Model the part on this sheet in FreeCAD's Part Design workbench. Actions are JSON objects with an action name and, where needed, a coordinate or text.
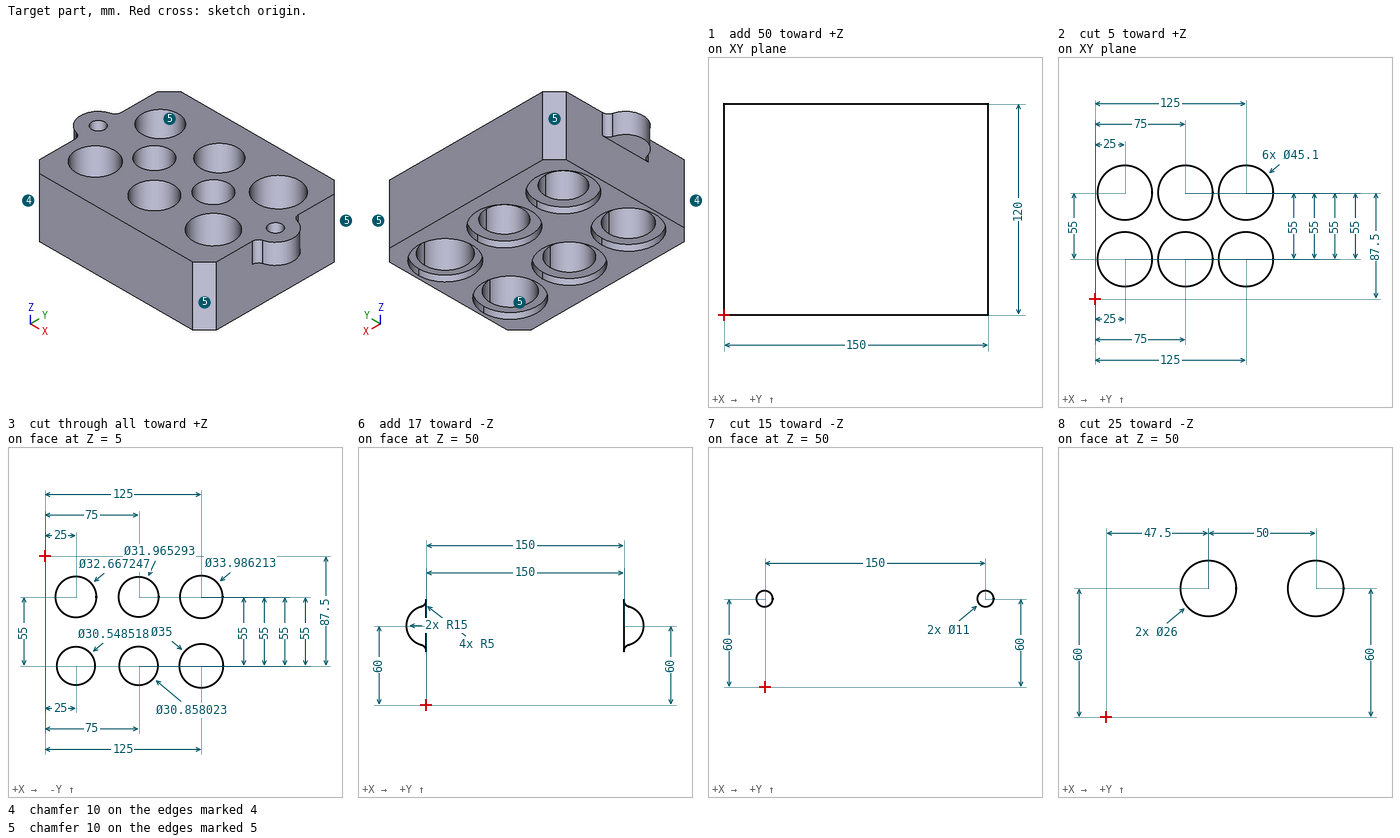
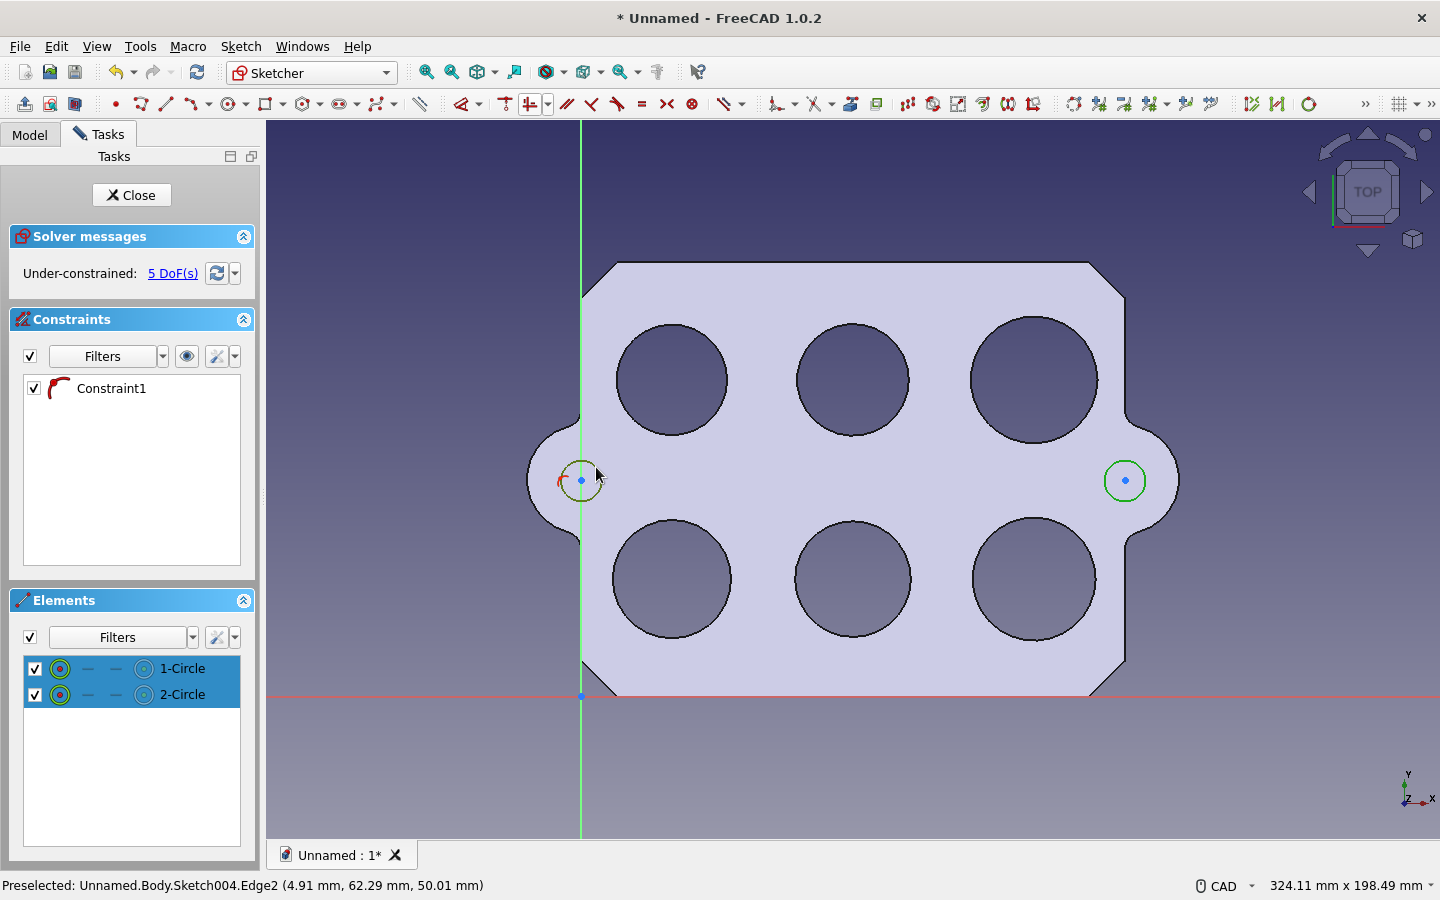
{"action": "left_click", "coordinate": [642, 104]}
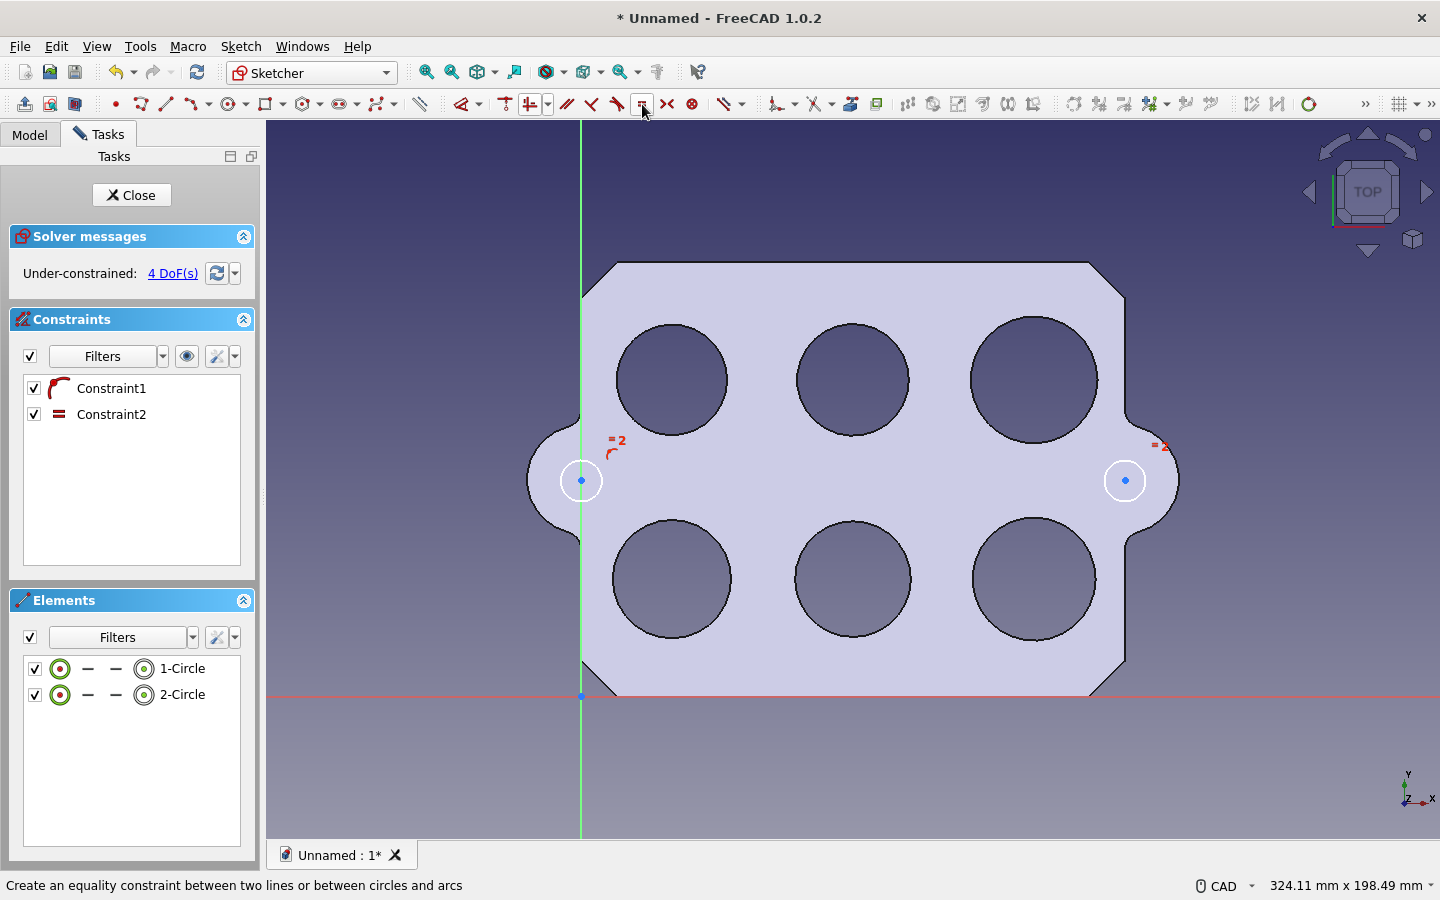
{"action": "key", "text": "d"}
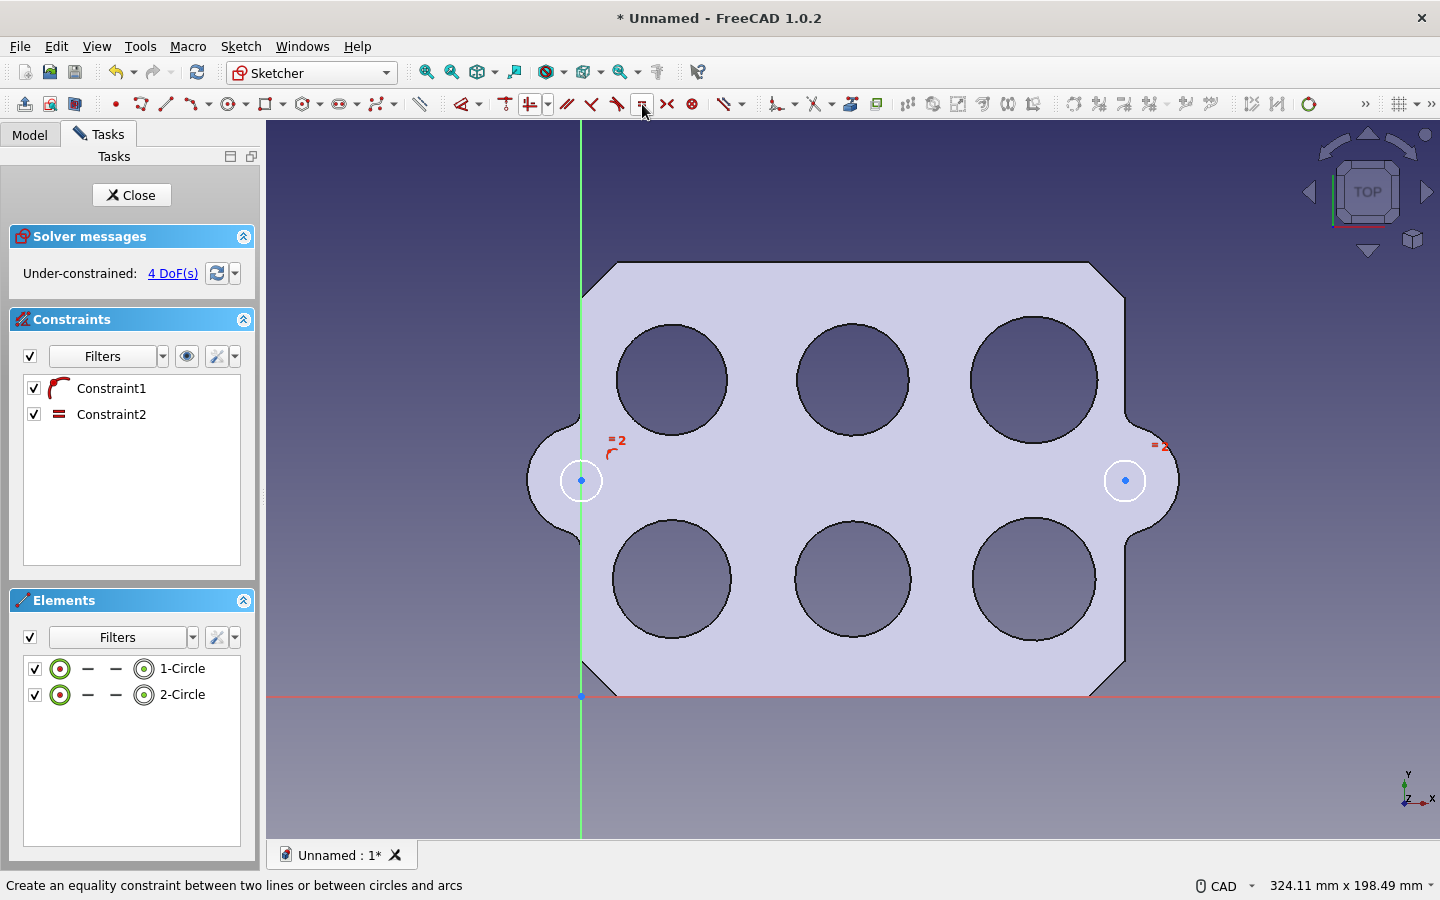
{"action": "left_click", "coordinate": [1139, 466]}
{"action": "left_click", "coordinate": [1161, 443]}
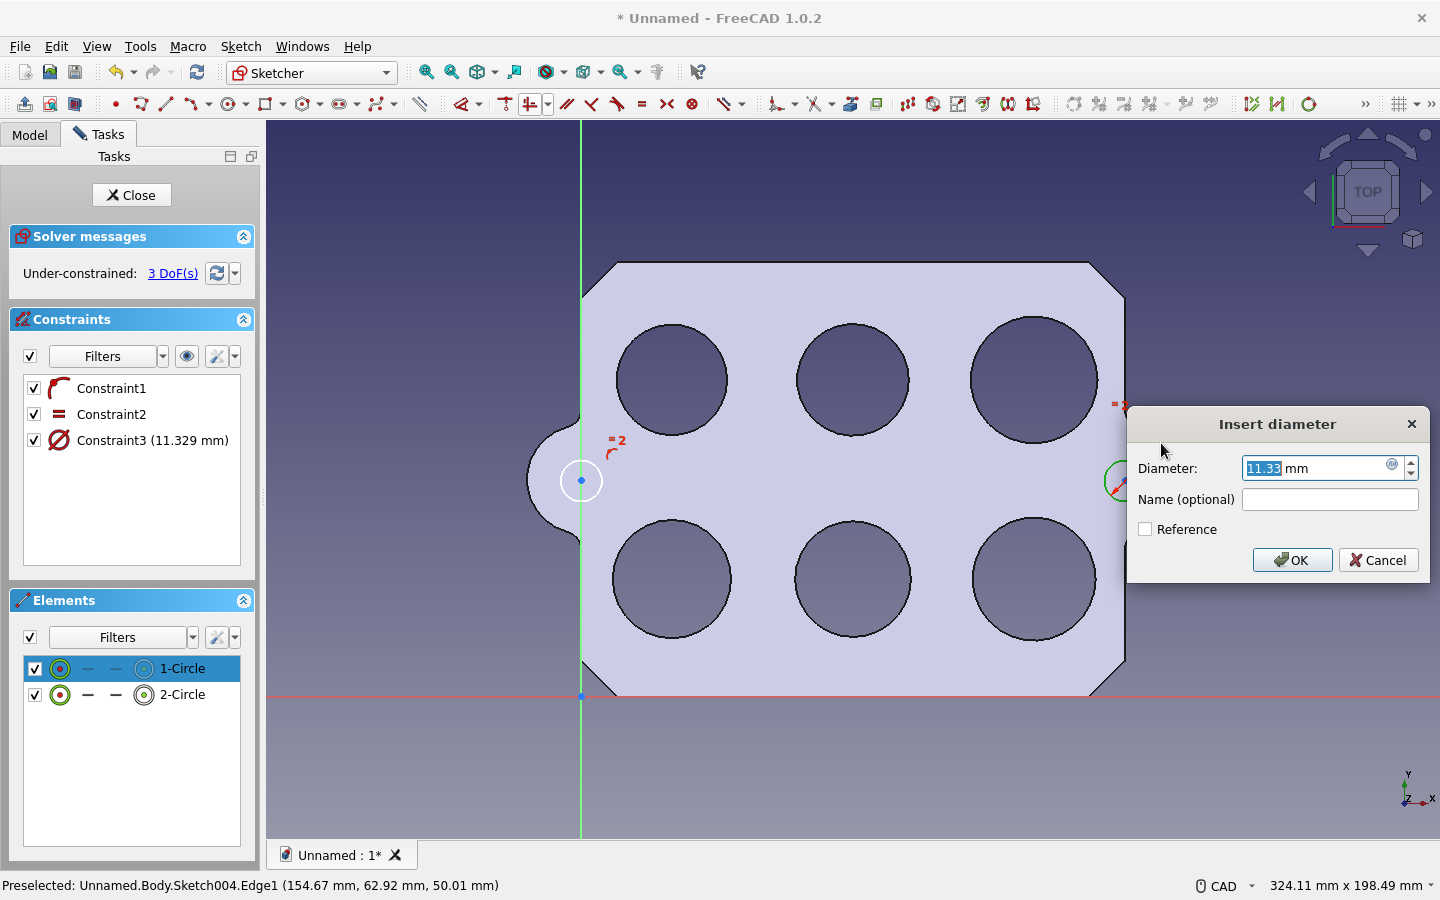
{"action": "type", "text": "11"}
{"action": "key", "text": "Return"}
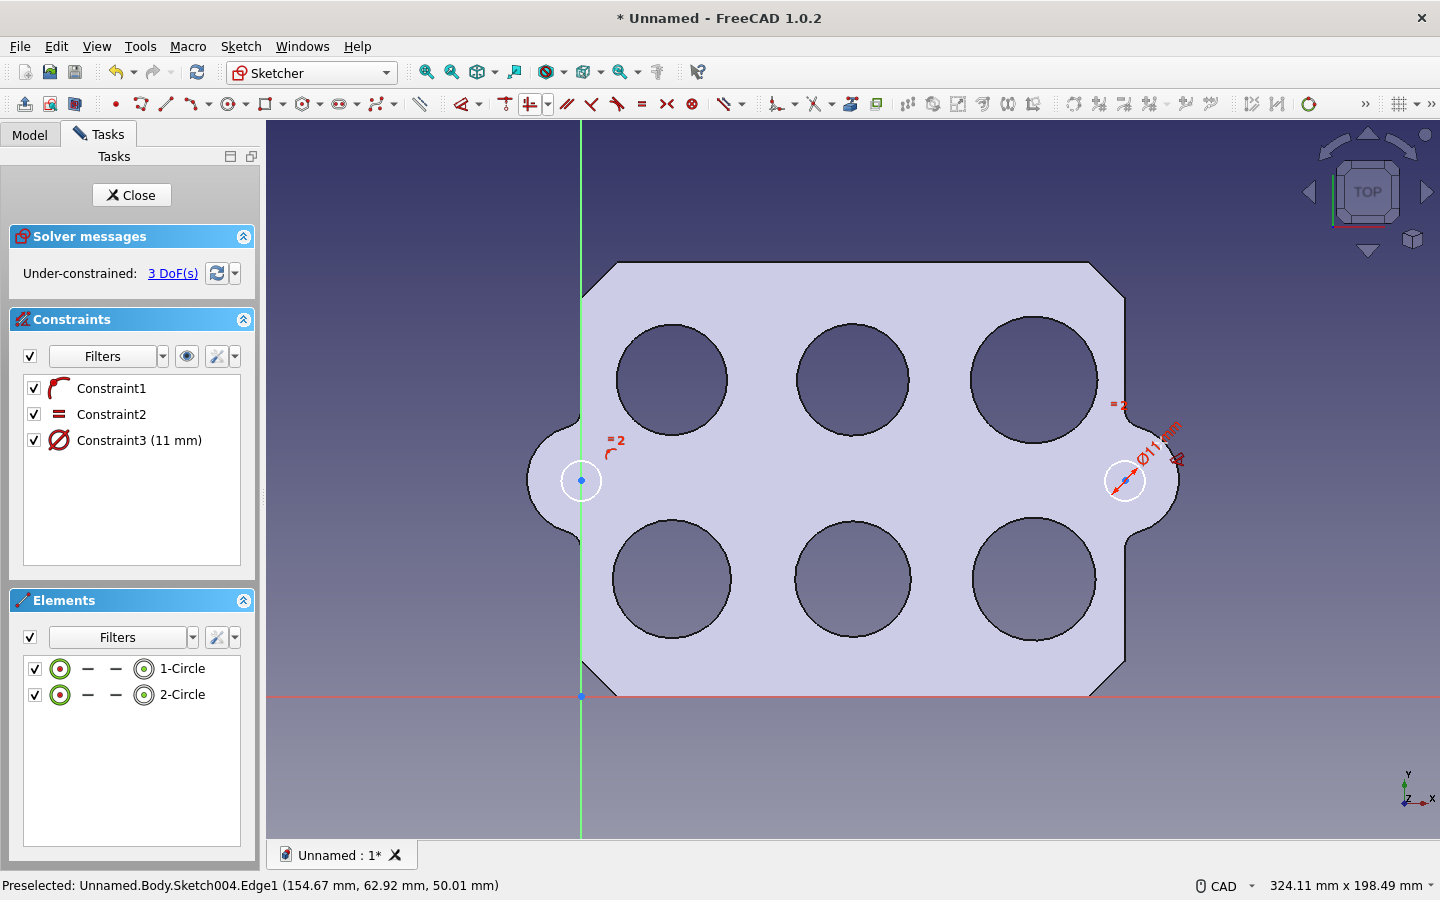
{"action": "left_click", "coordinate": [1125, 481]}
{"action": "left_click", "coordinate": [1159, 589]}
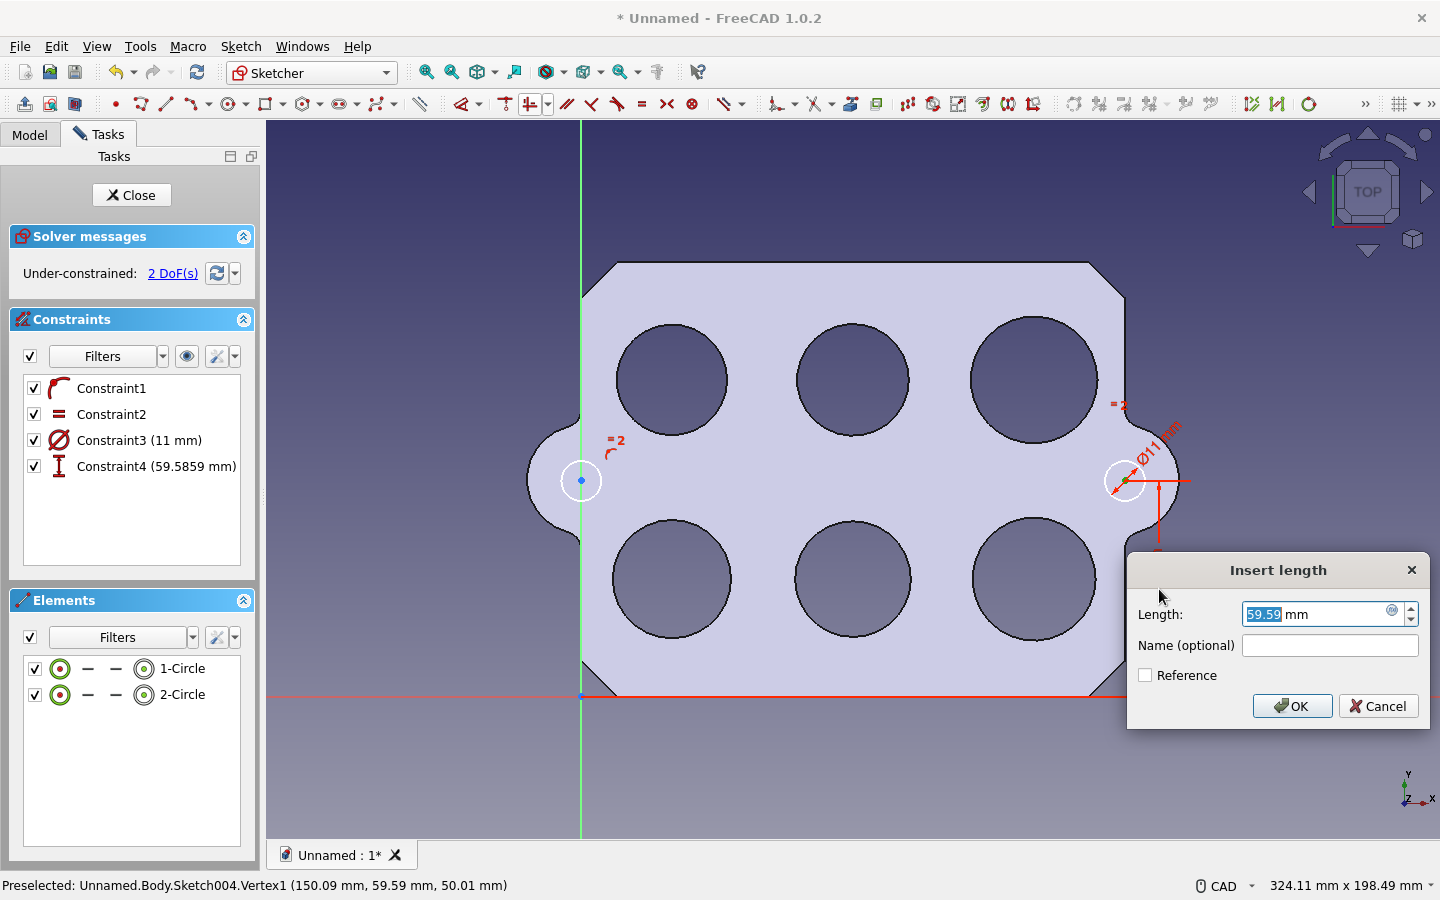
{"action": "type", "text": "60"}
{"action": "key", "text": "Return"}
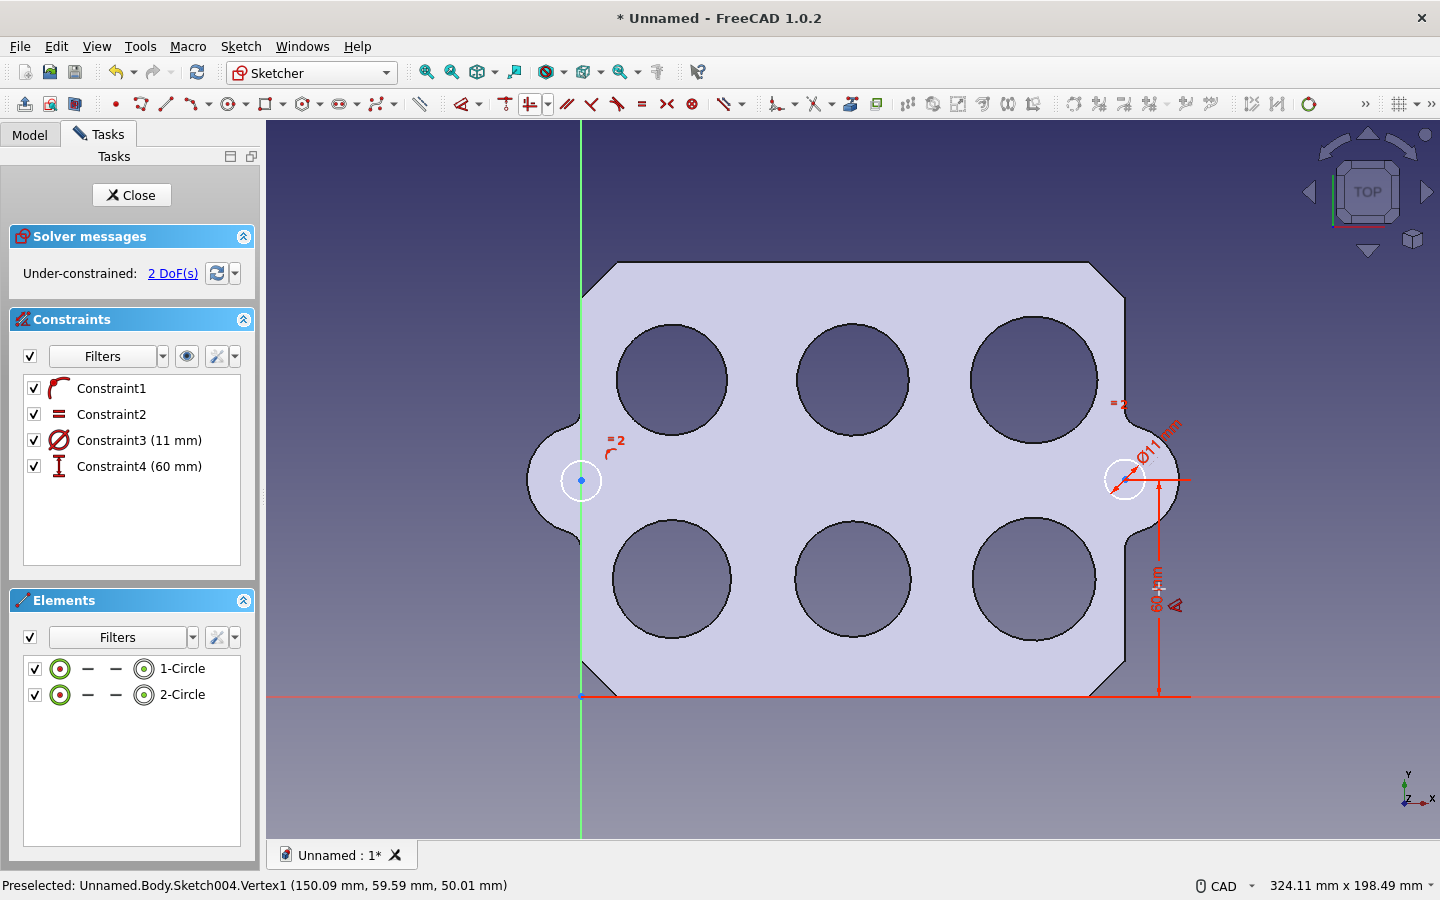
{"action": "left_click", "coordinate": [581, 481]}
{"action": "left_click", "coordinate": [547, 589]}